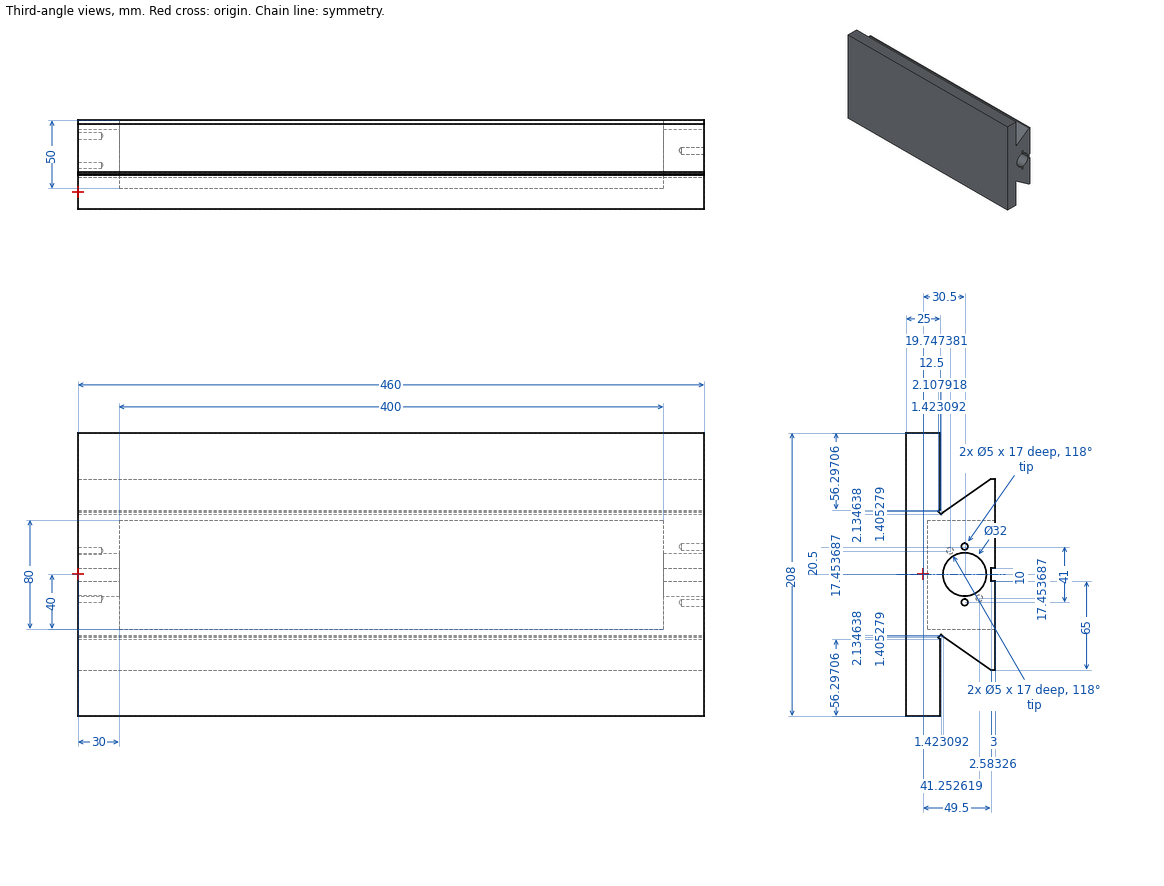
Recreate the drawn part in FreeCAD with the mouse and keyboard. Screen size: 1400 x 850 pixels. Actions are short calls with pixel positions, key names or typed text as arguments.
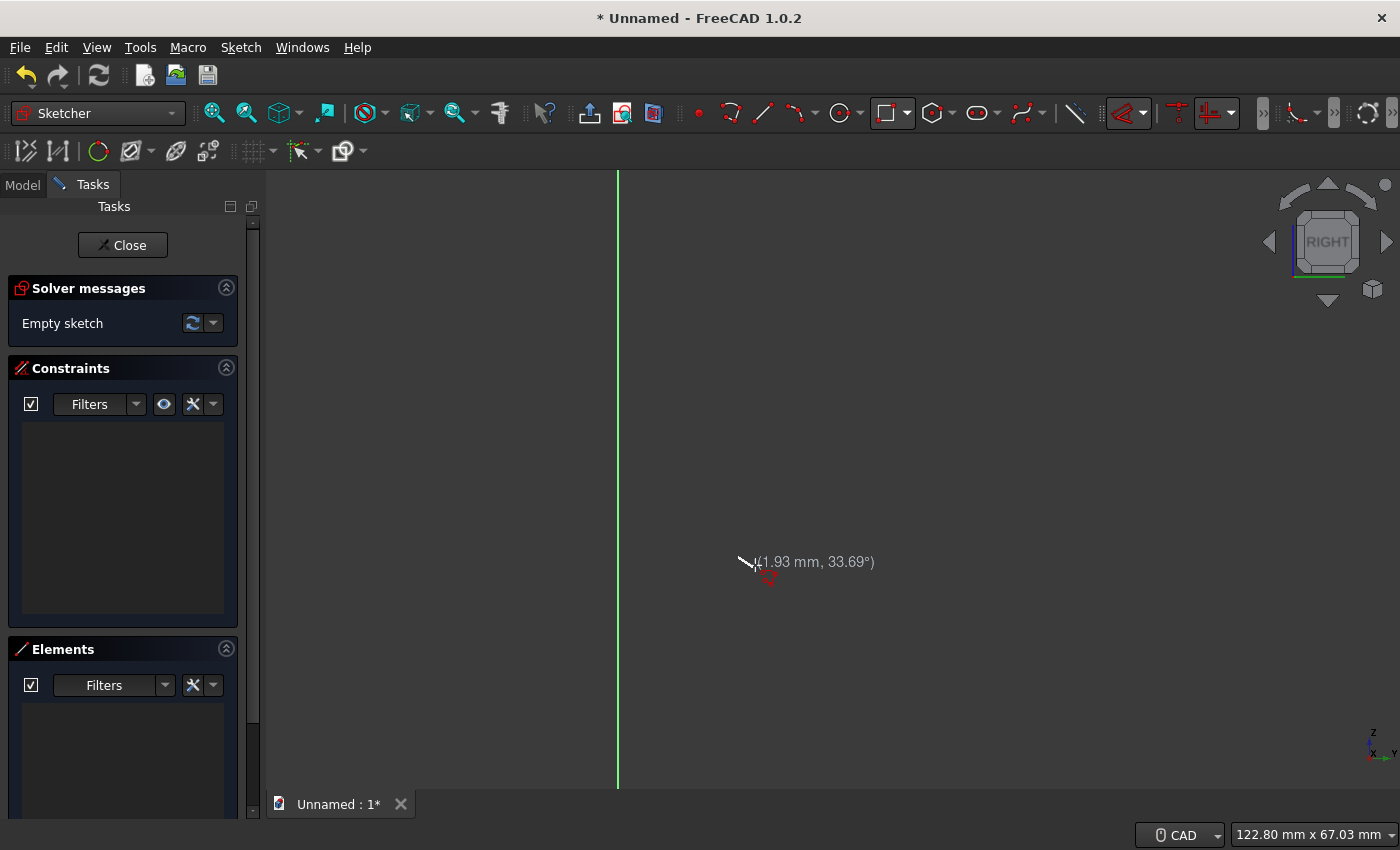
click(753, 563)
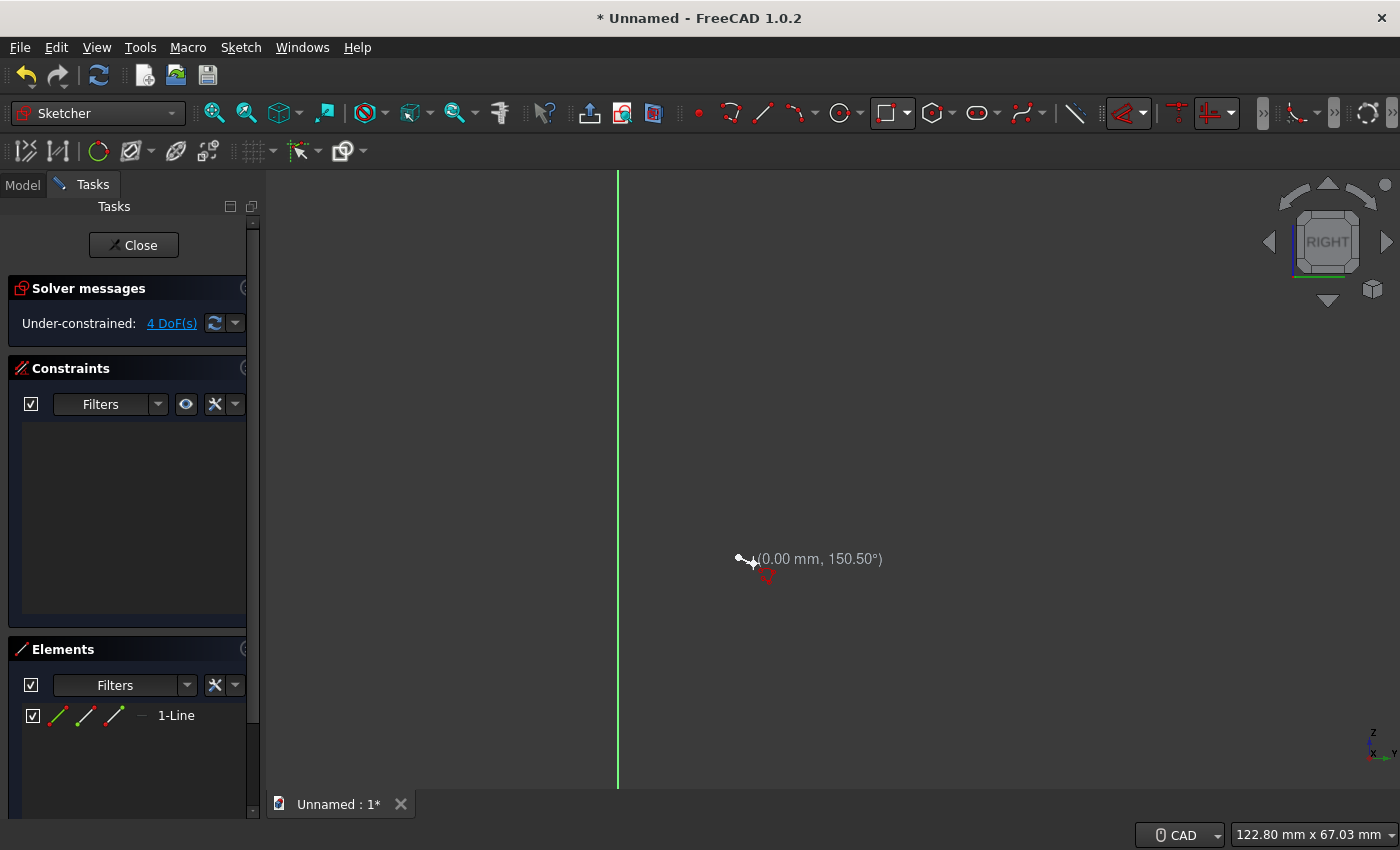
scroll(755, 565, down, 8)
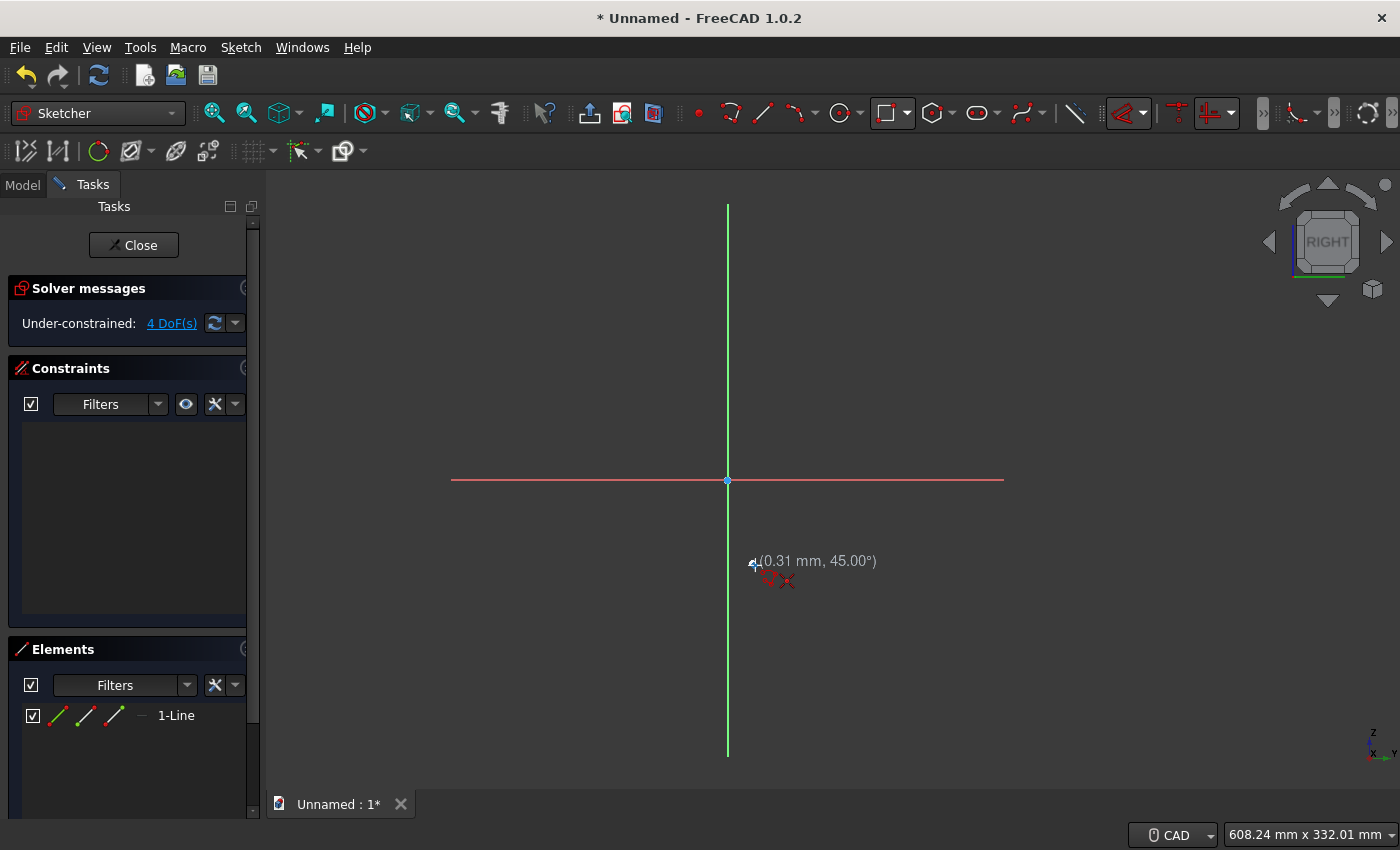
click(820, 611)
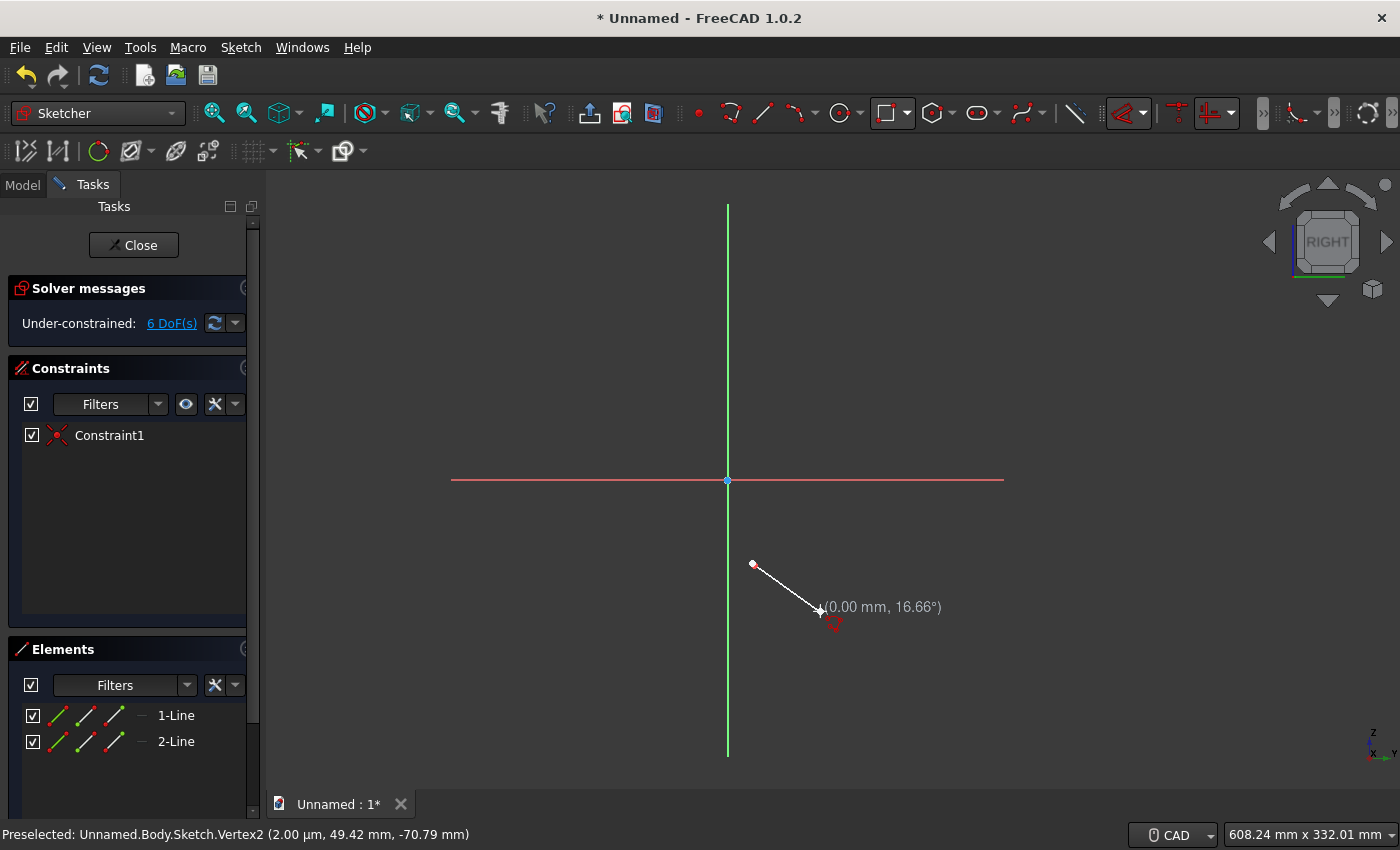
scroll(826, 611, up, 6)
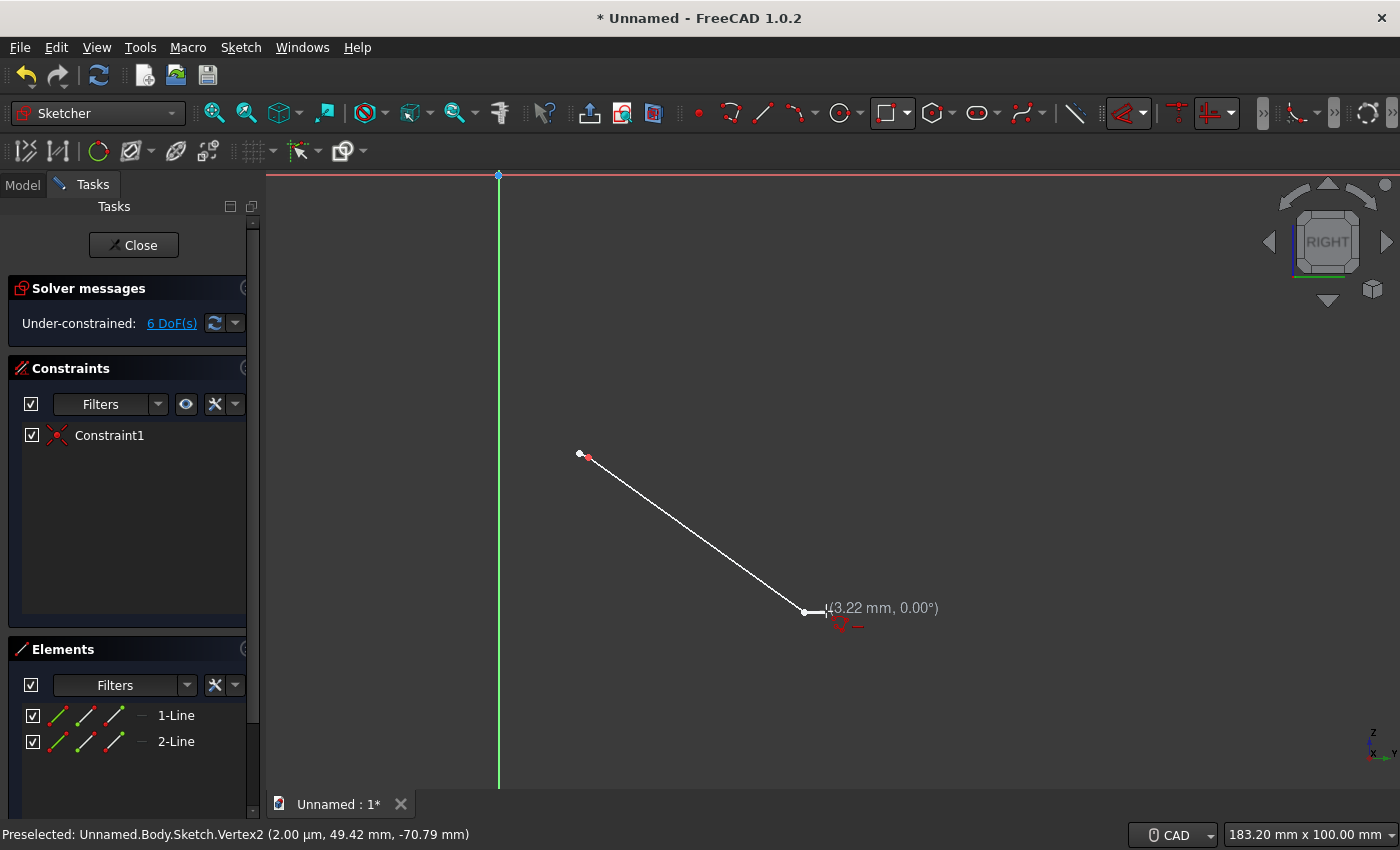
click(824, 609)
click(824, 206)
click(808, 206)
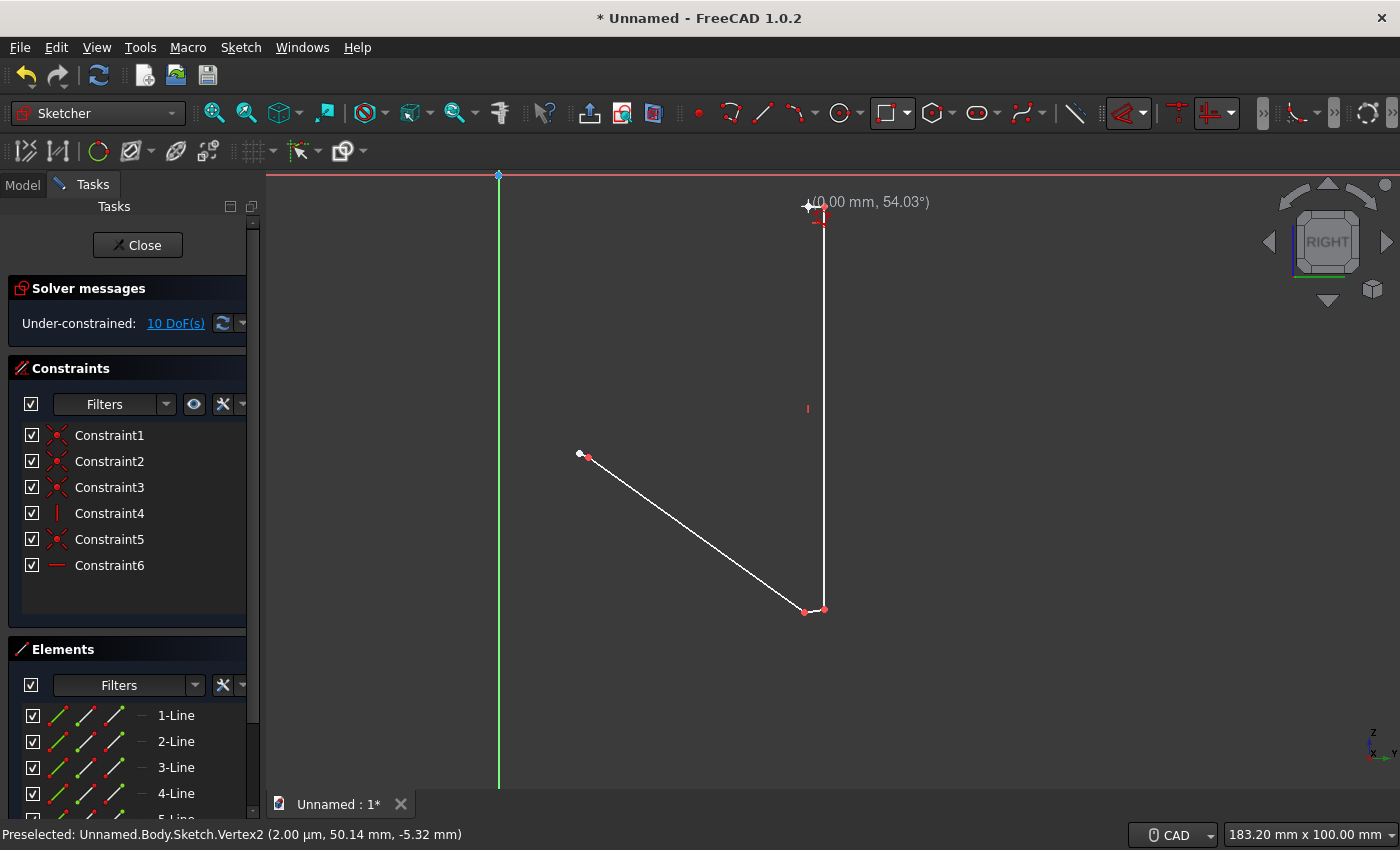
scroll(826, 611, down, 6)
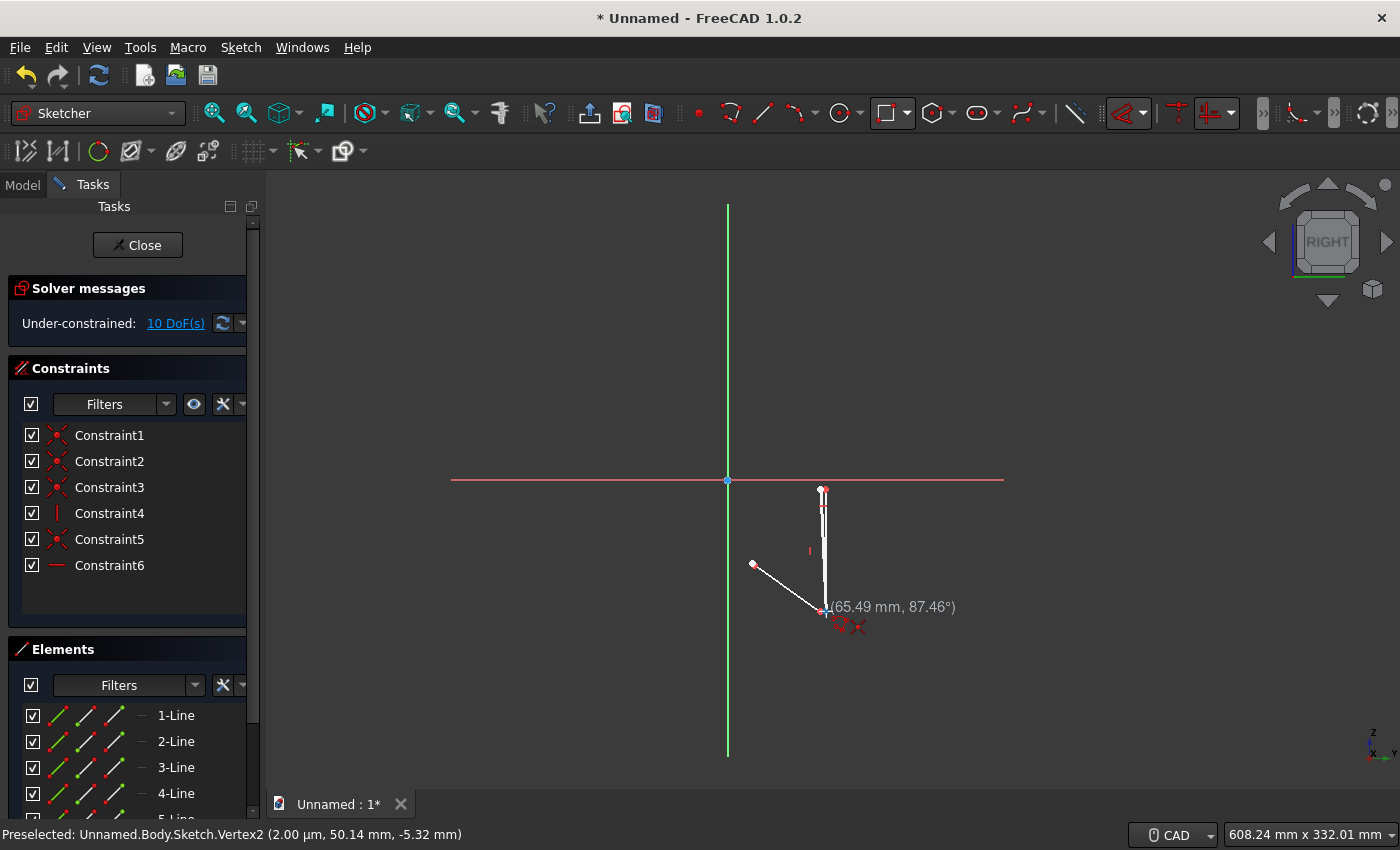
scroll(821, 471, up, 3)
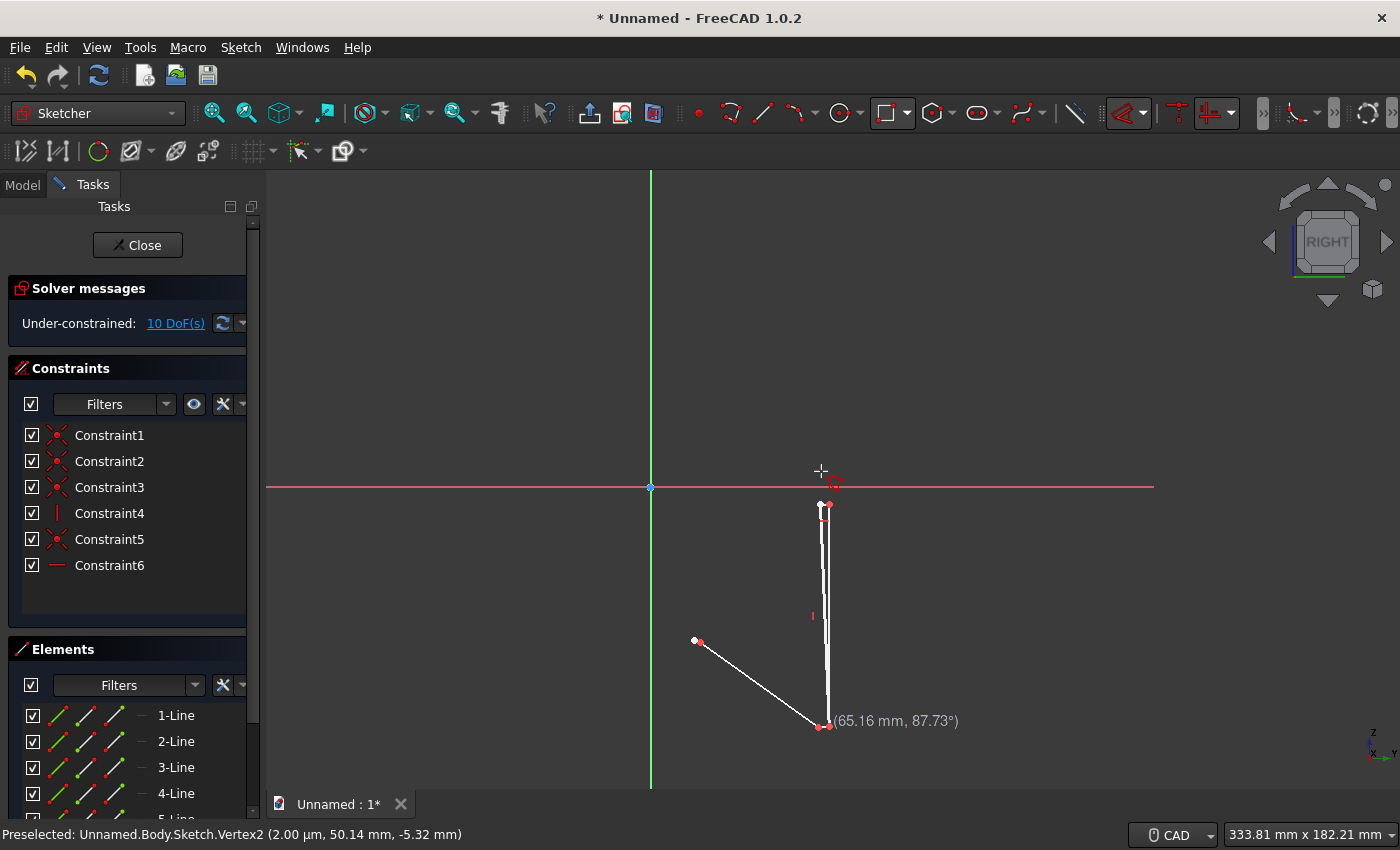
click(820, 470)